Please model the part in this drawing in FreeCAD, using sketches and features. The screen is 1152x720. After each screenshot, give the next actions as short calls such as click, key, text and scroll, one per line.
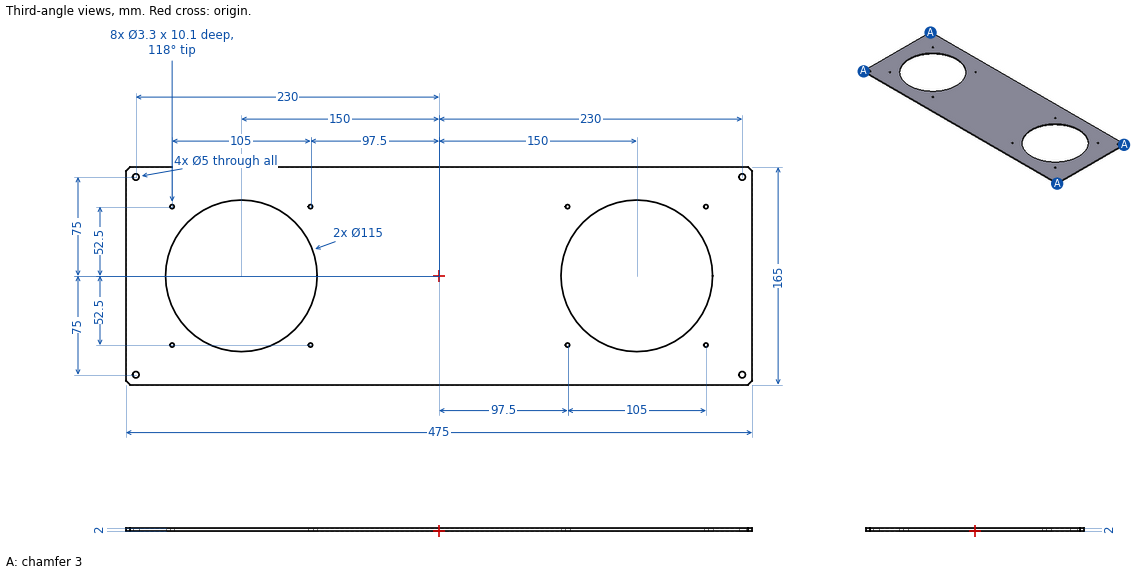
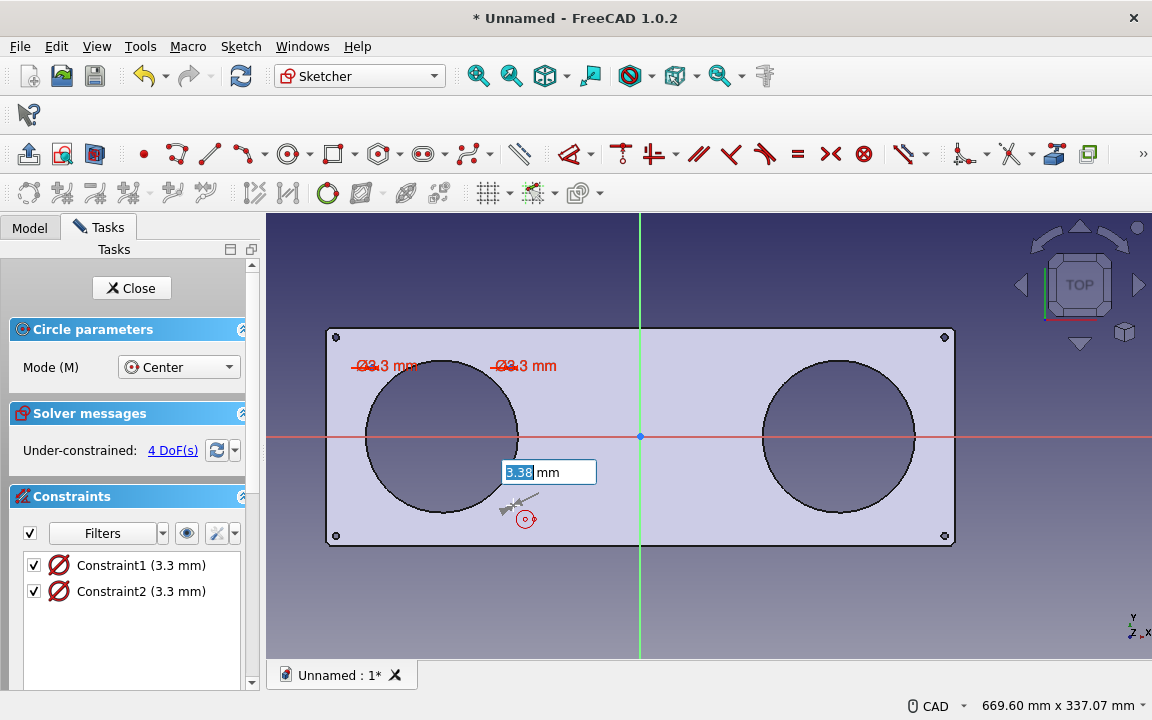
text(3.3)
key(Return)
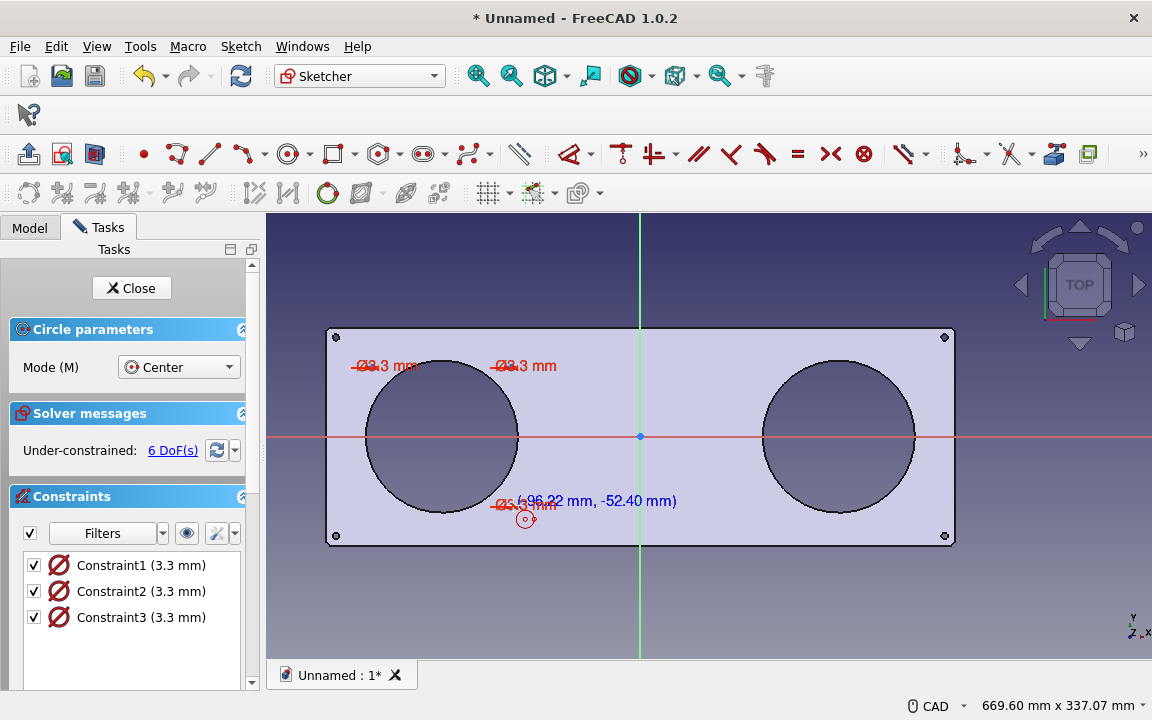
scroll(372, 506, up, 12)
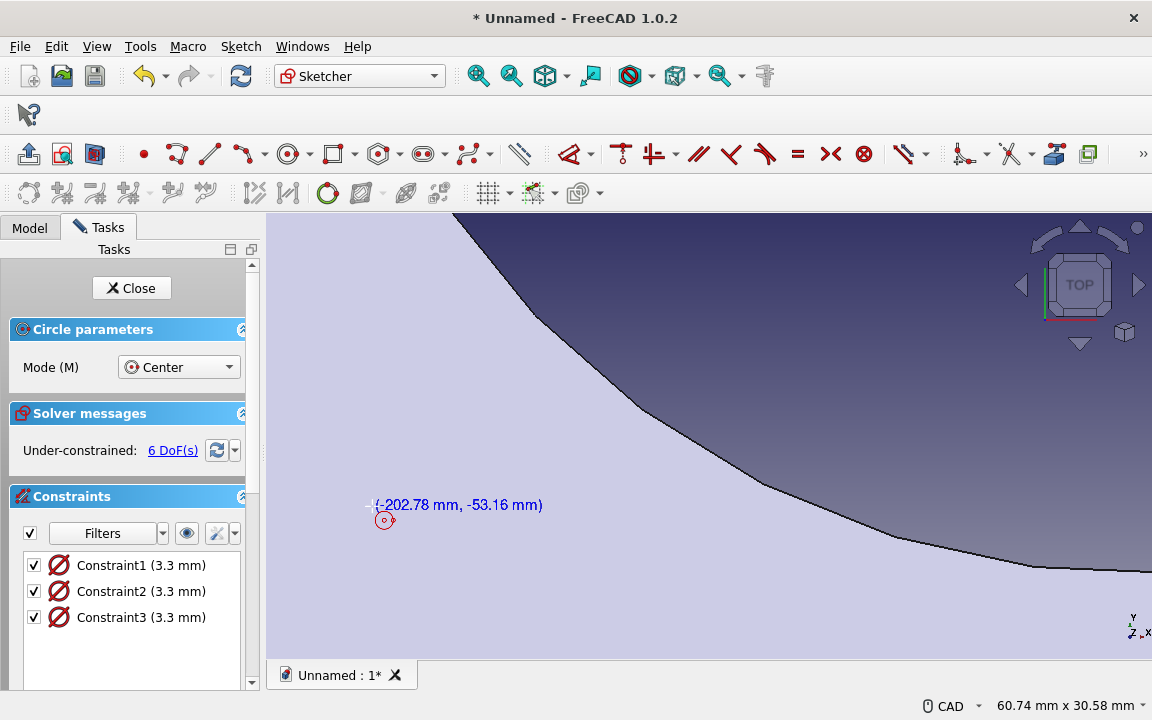
scroll(372, 506, down, 12)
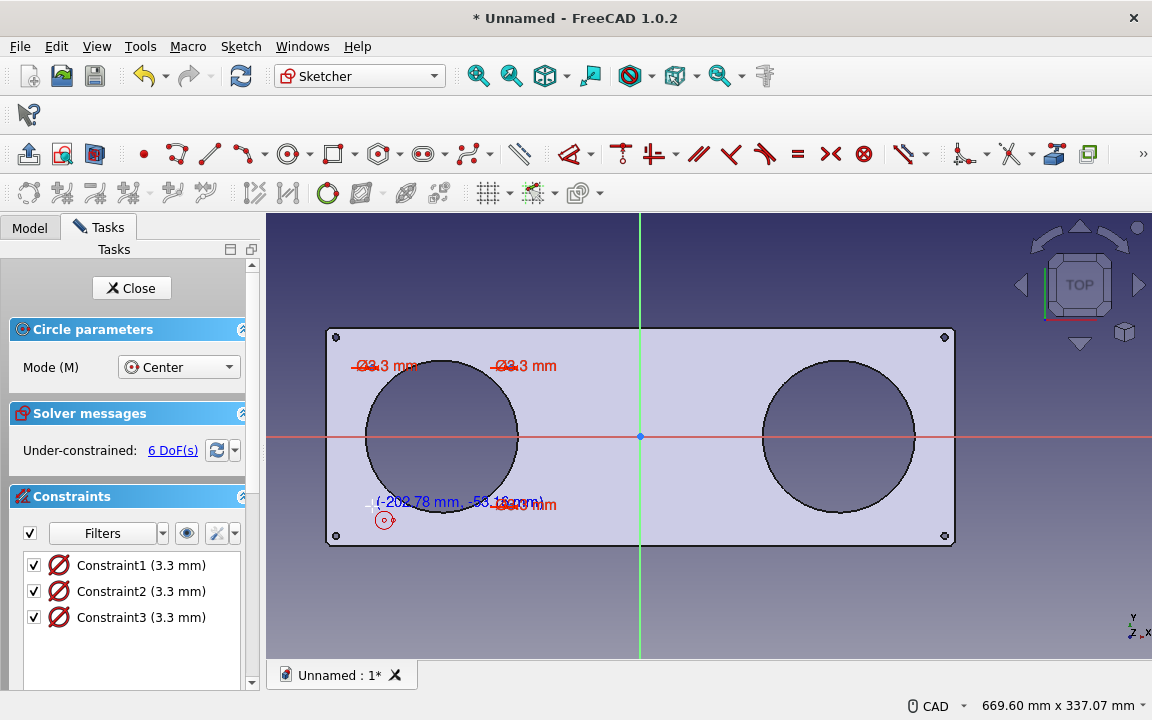
click(372, 506)
move(374, 505)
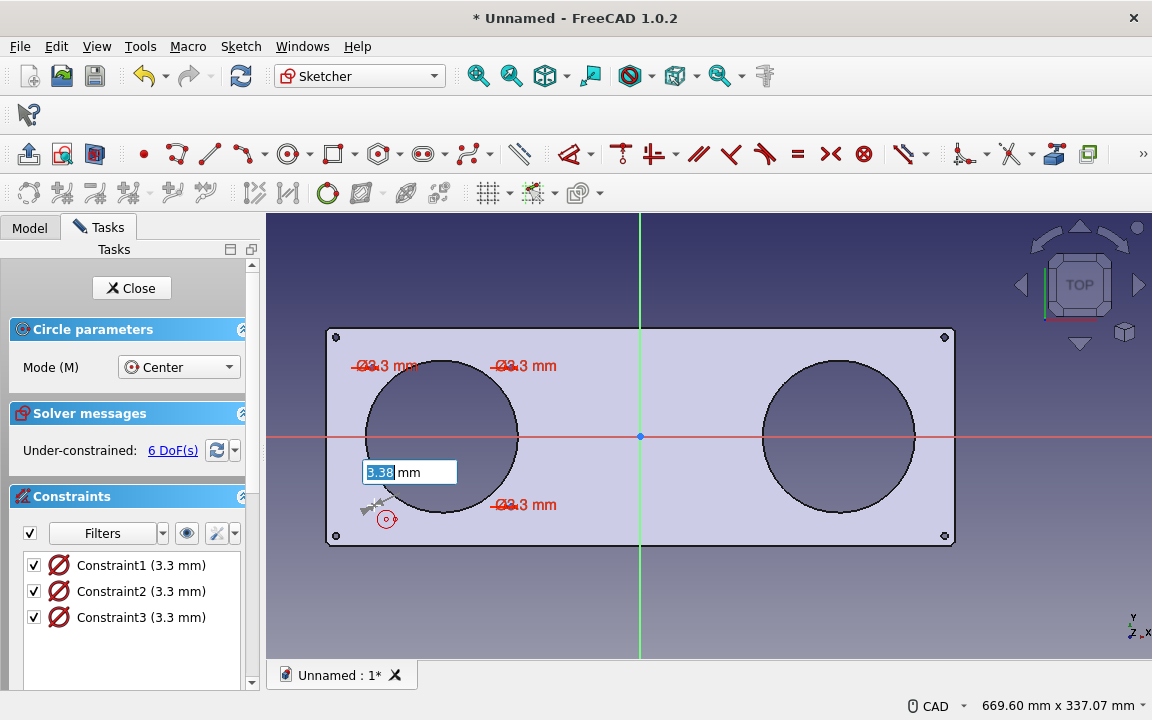
text(3.3)
key(Return)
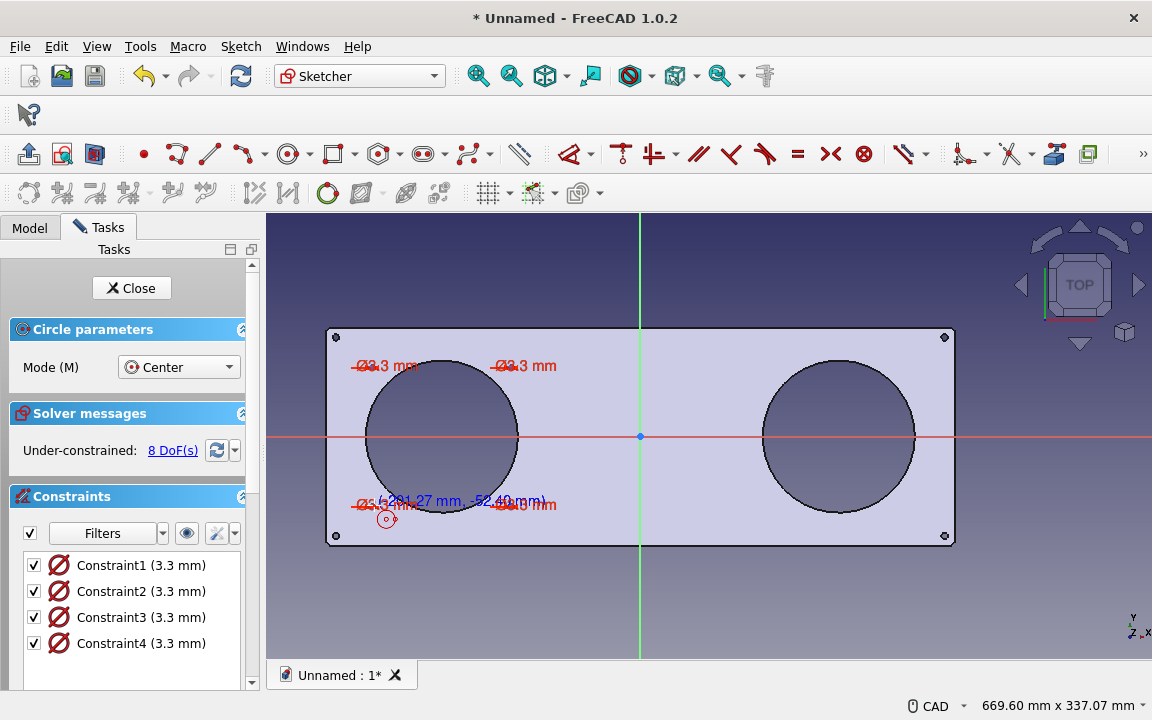
scroll(769, 506, up, 12)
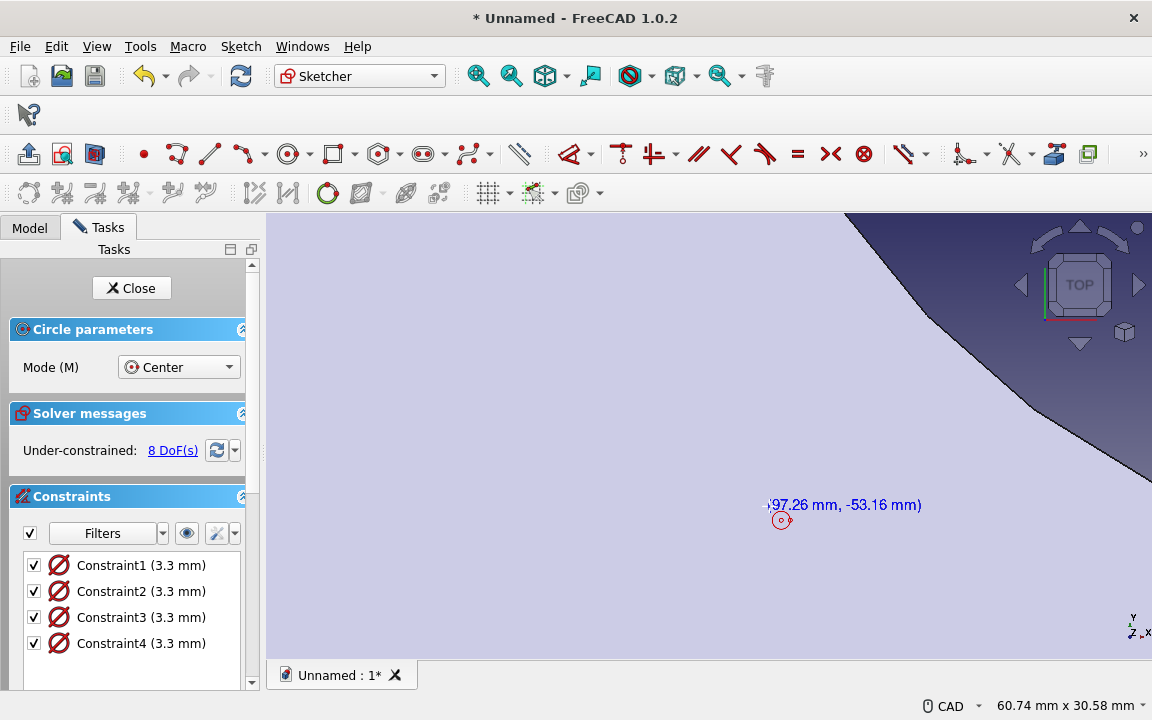
scroll(770, 506, down, 12)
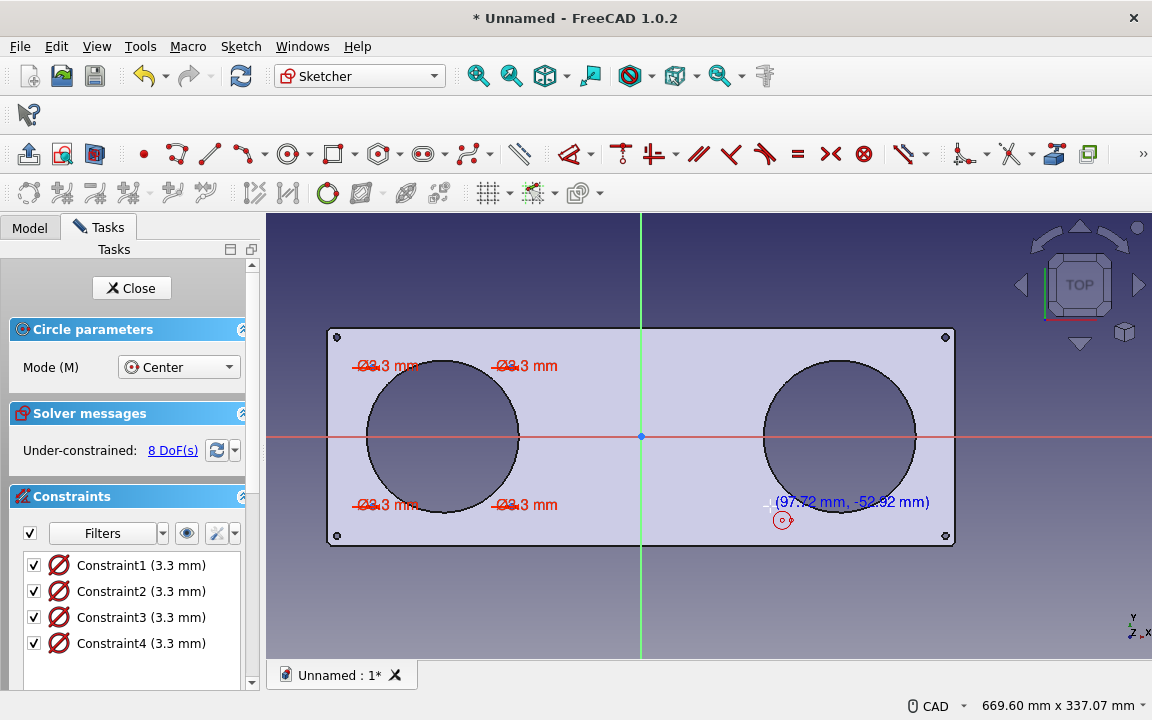
click(770, 506)
move(772, 505)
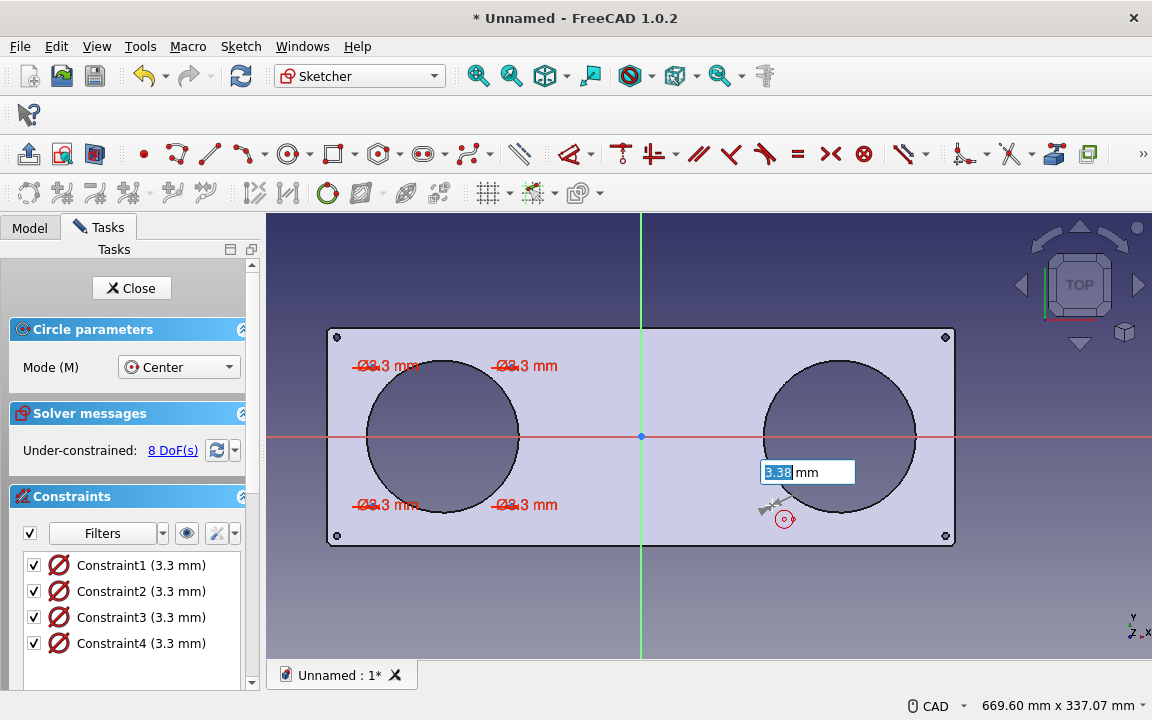
text(3.3)
key(Return)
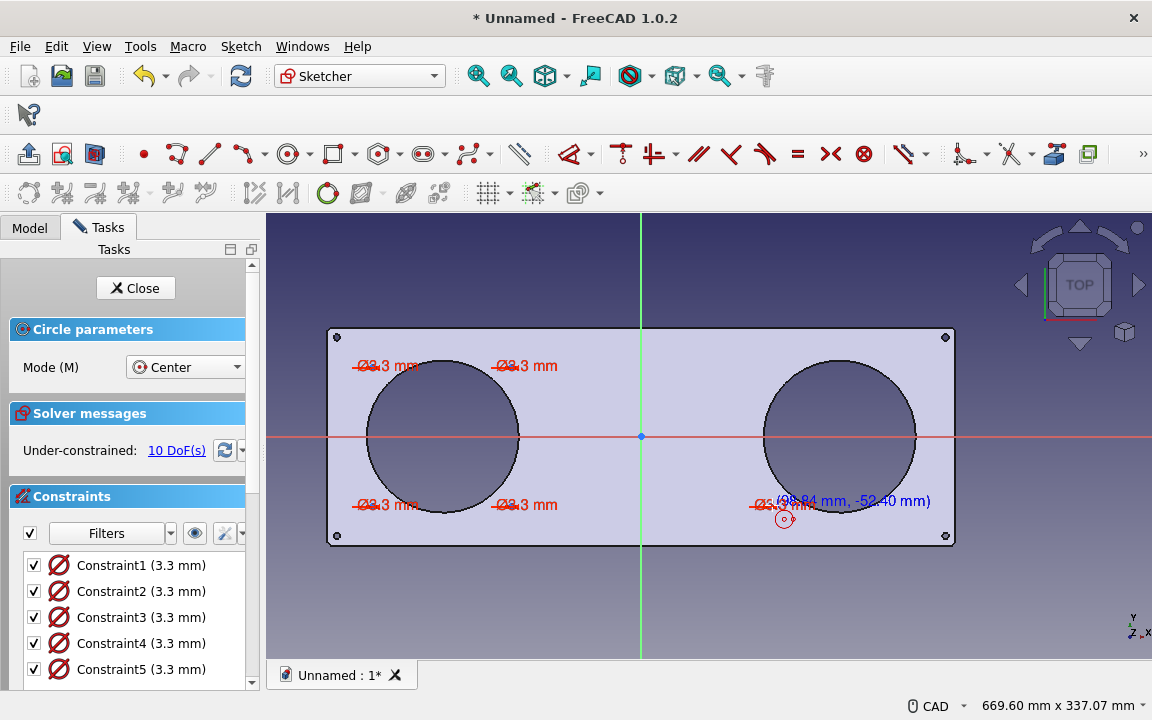
scroll(909, 506, up, 12)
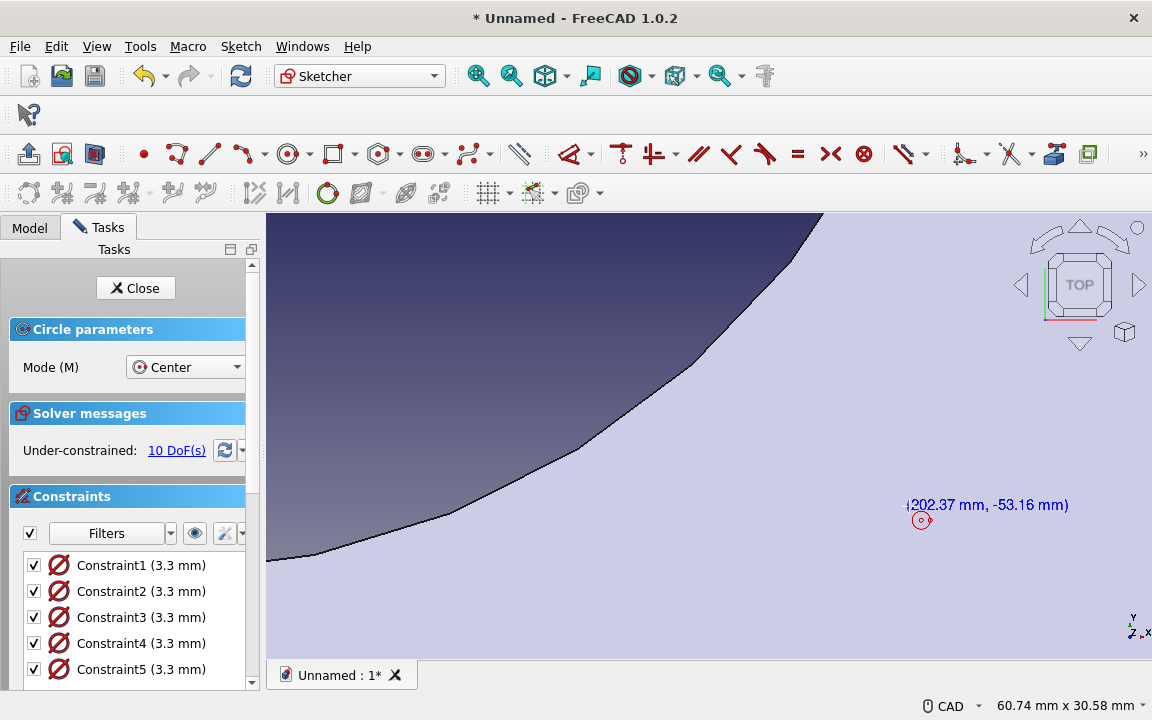
scroll(909, 506, down, 12)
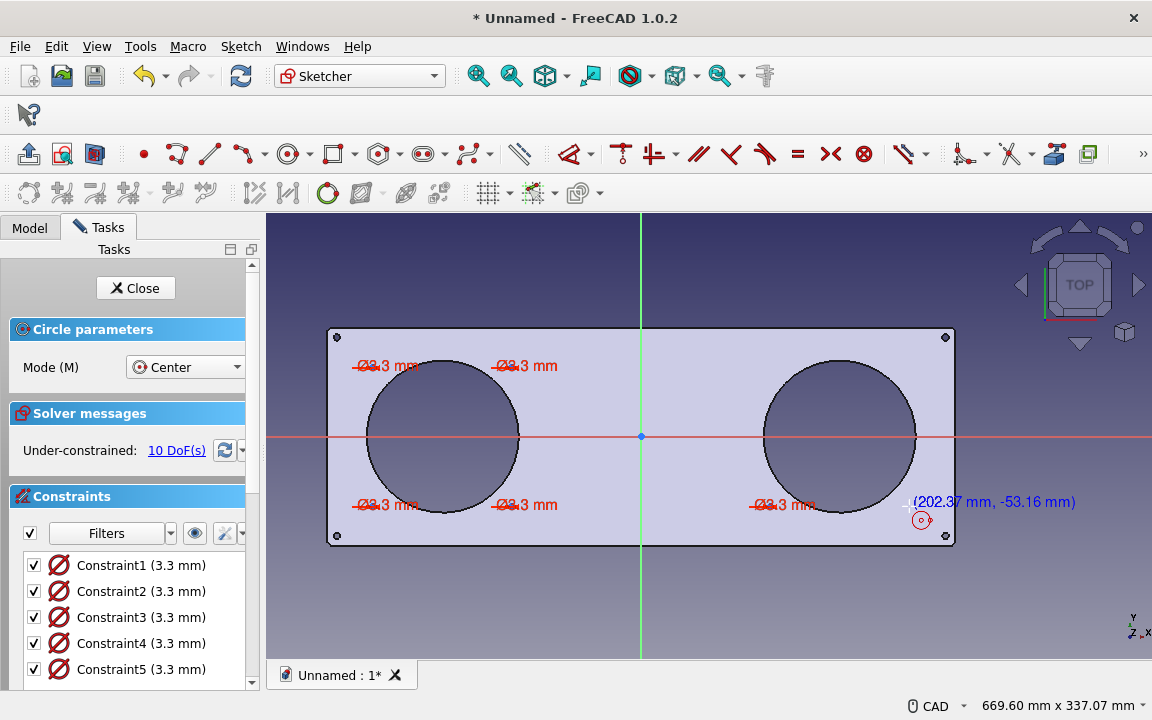
click(909, 506)
move(911, 505)